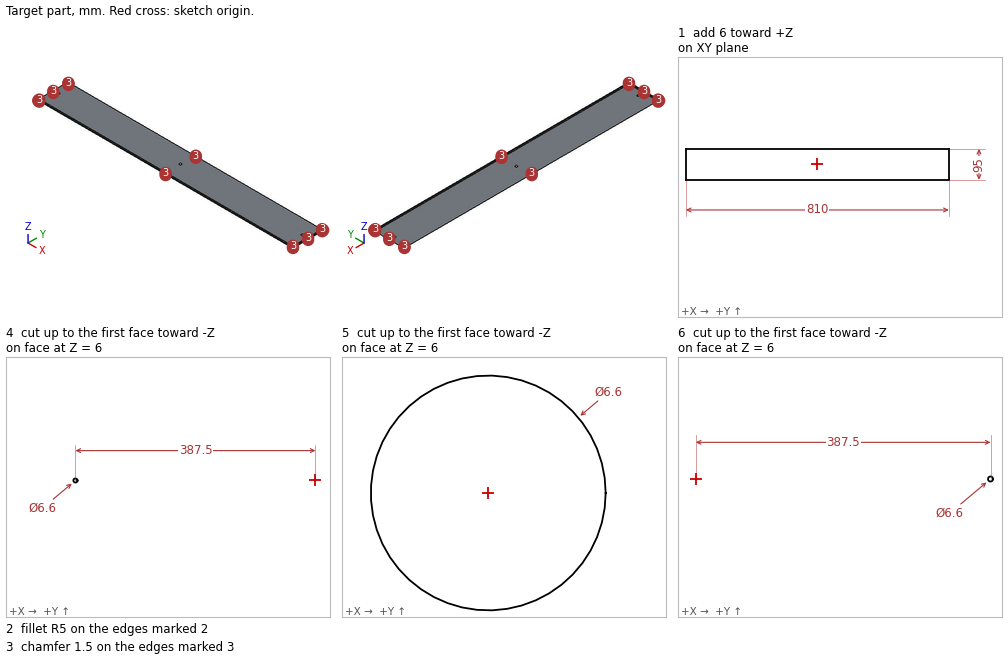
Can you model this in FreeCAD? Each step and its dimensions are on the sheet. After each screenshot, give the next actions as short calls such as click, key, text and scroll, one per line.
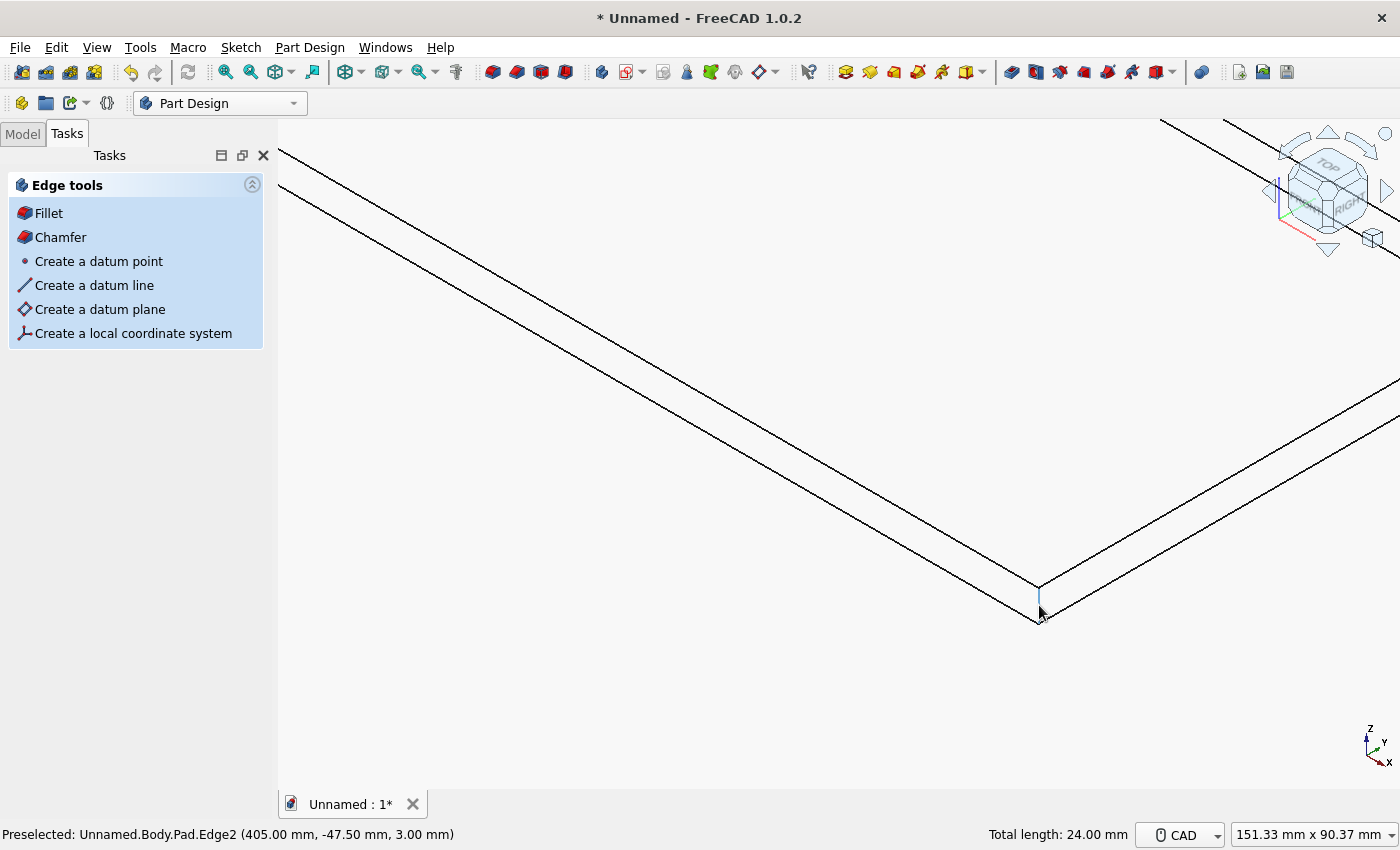
key(v)
key(1)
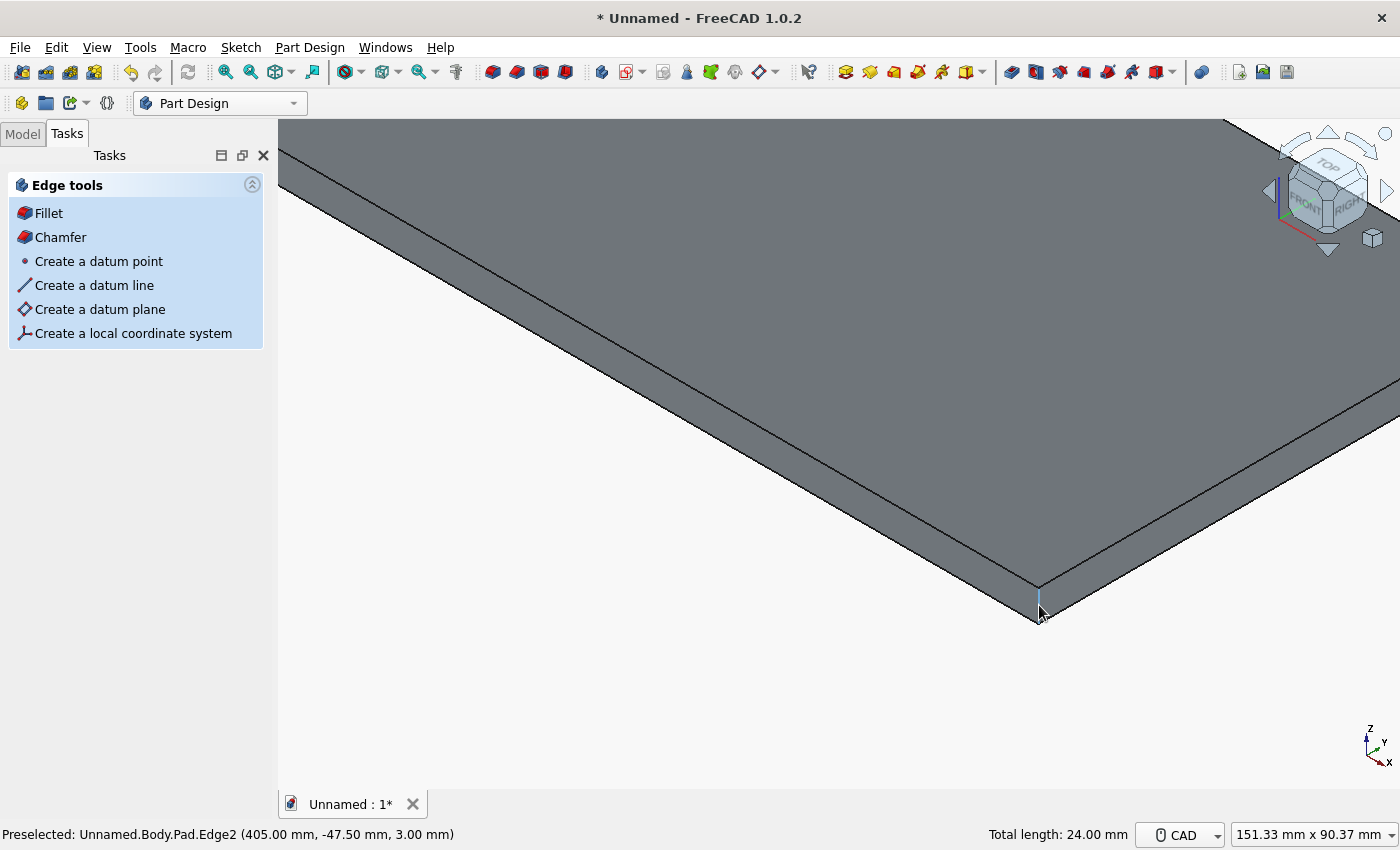
click(494, 72)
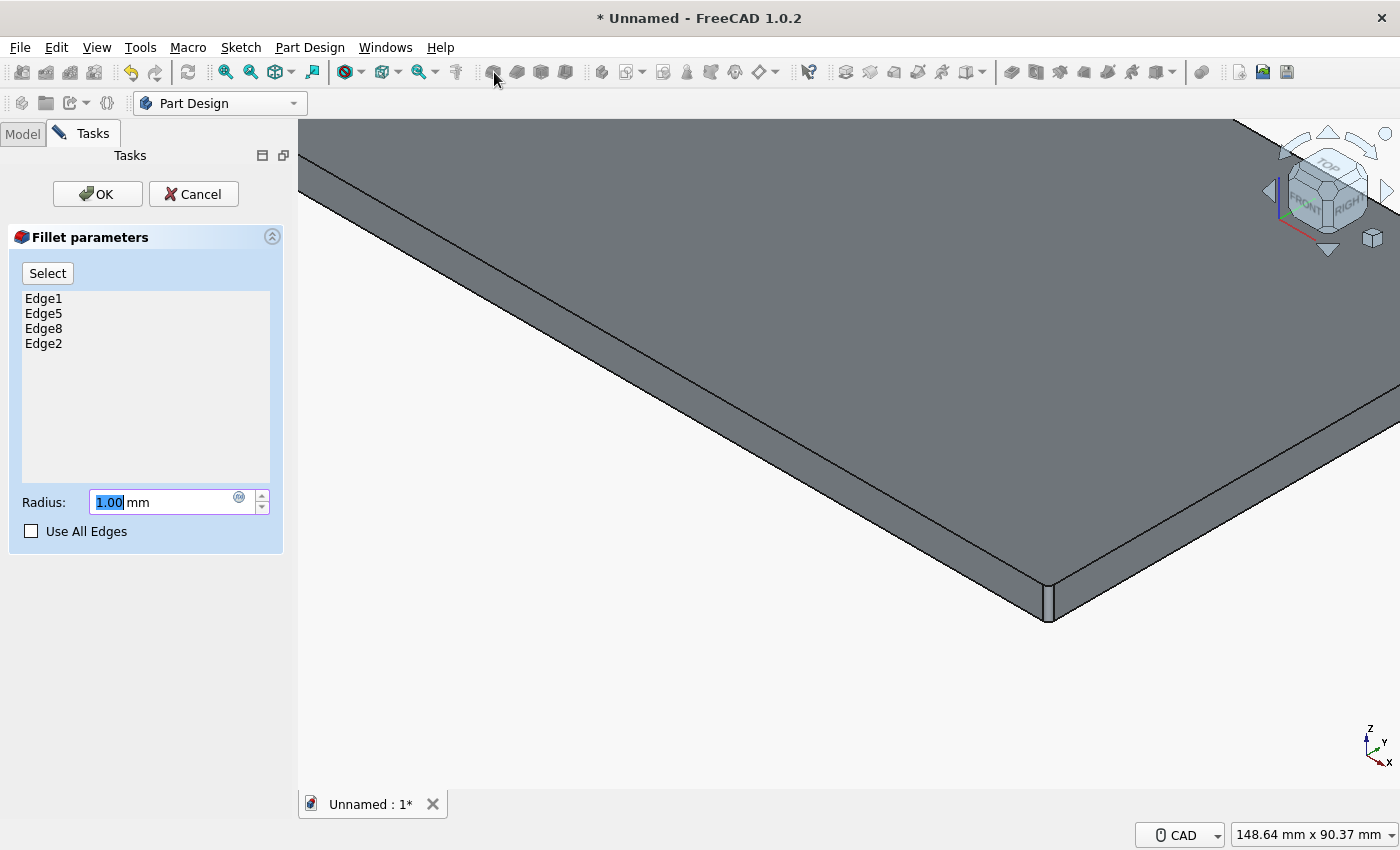
text(5)
key(Tab)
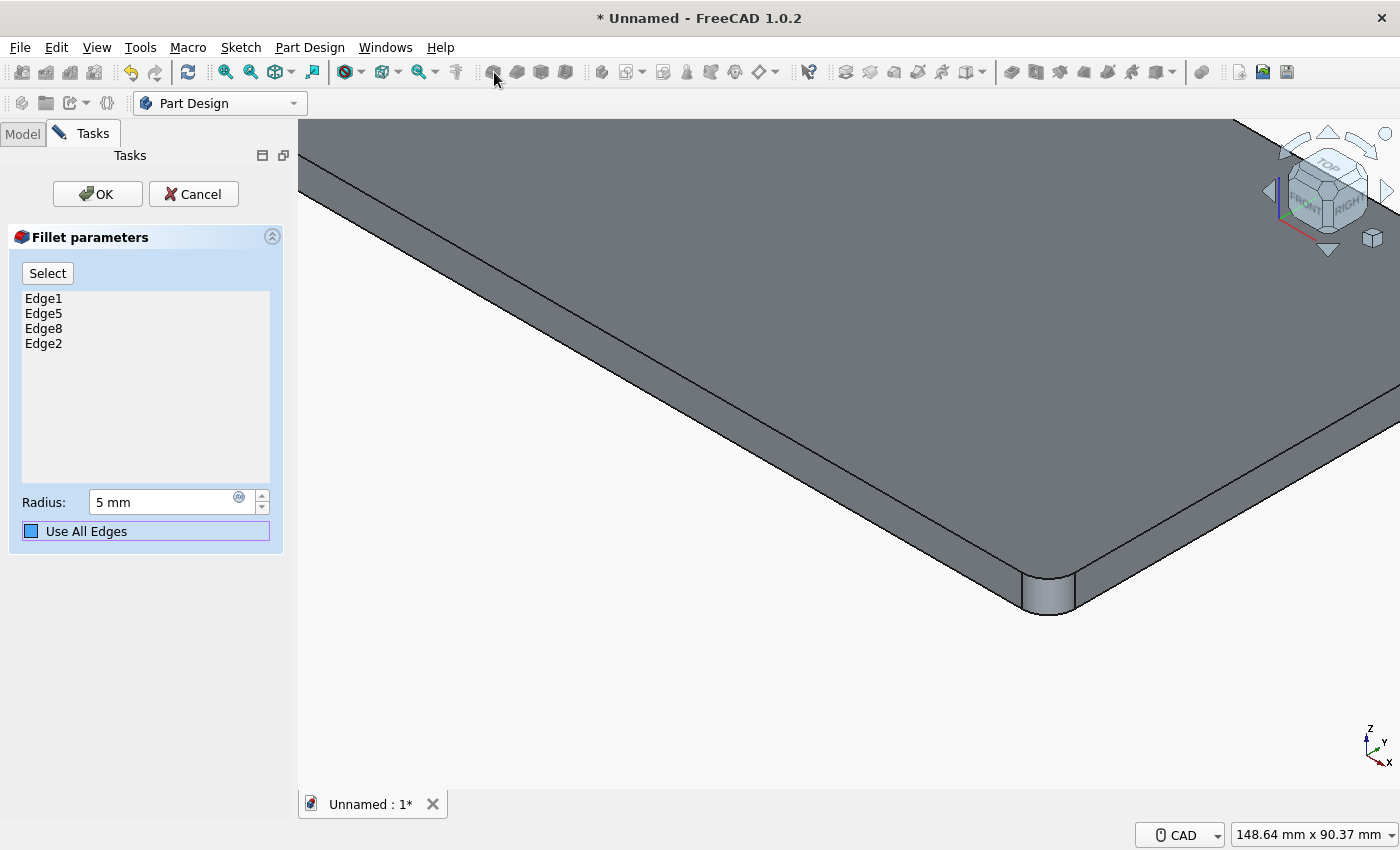
click(98, 194)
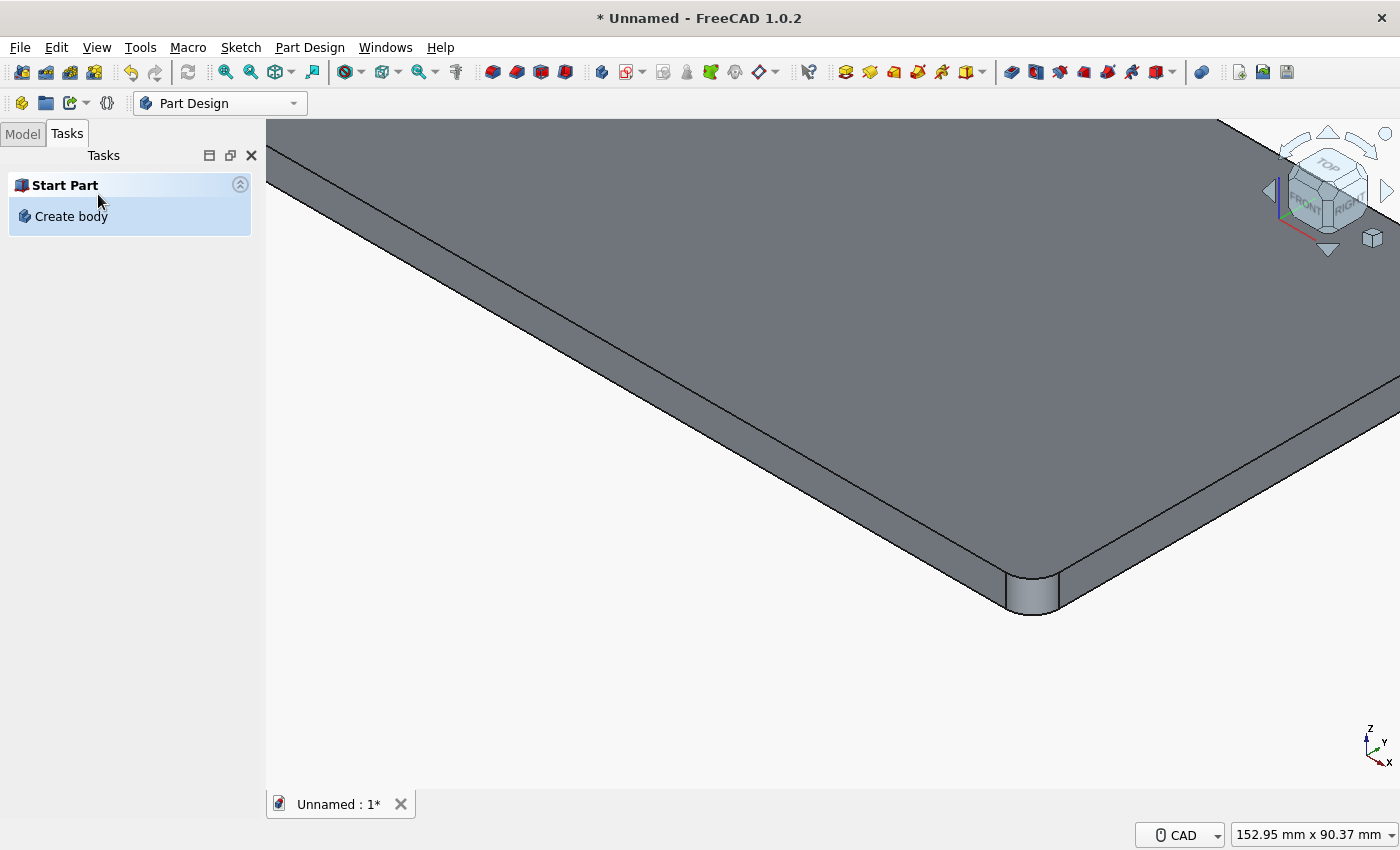
key(v)
key(f)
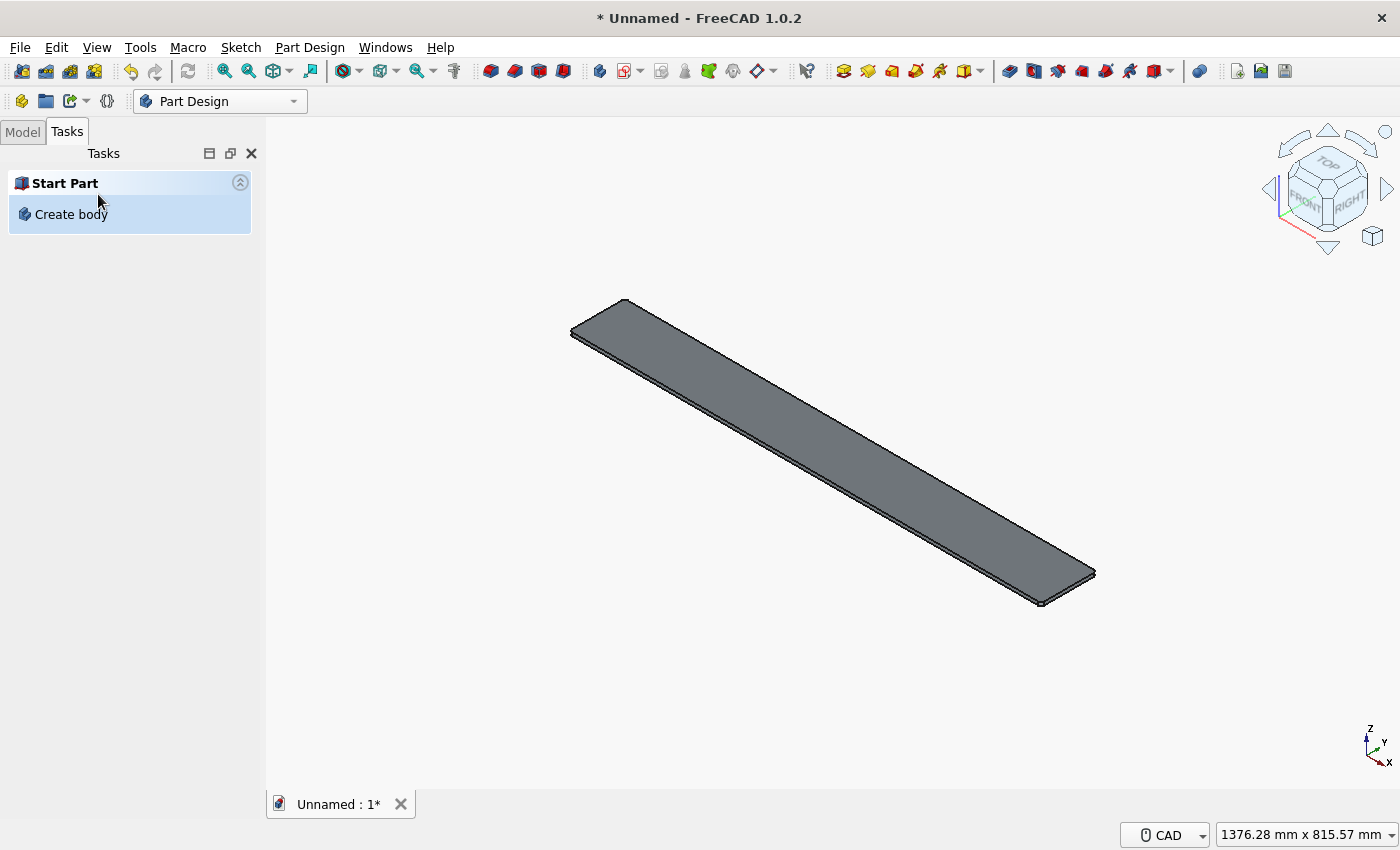
click(1035, 567)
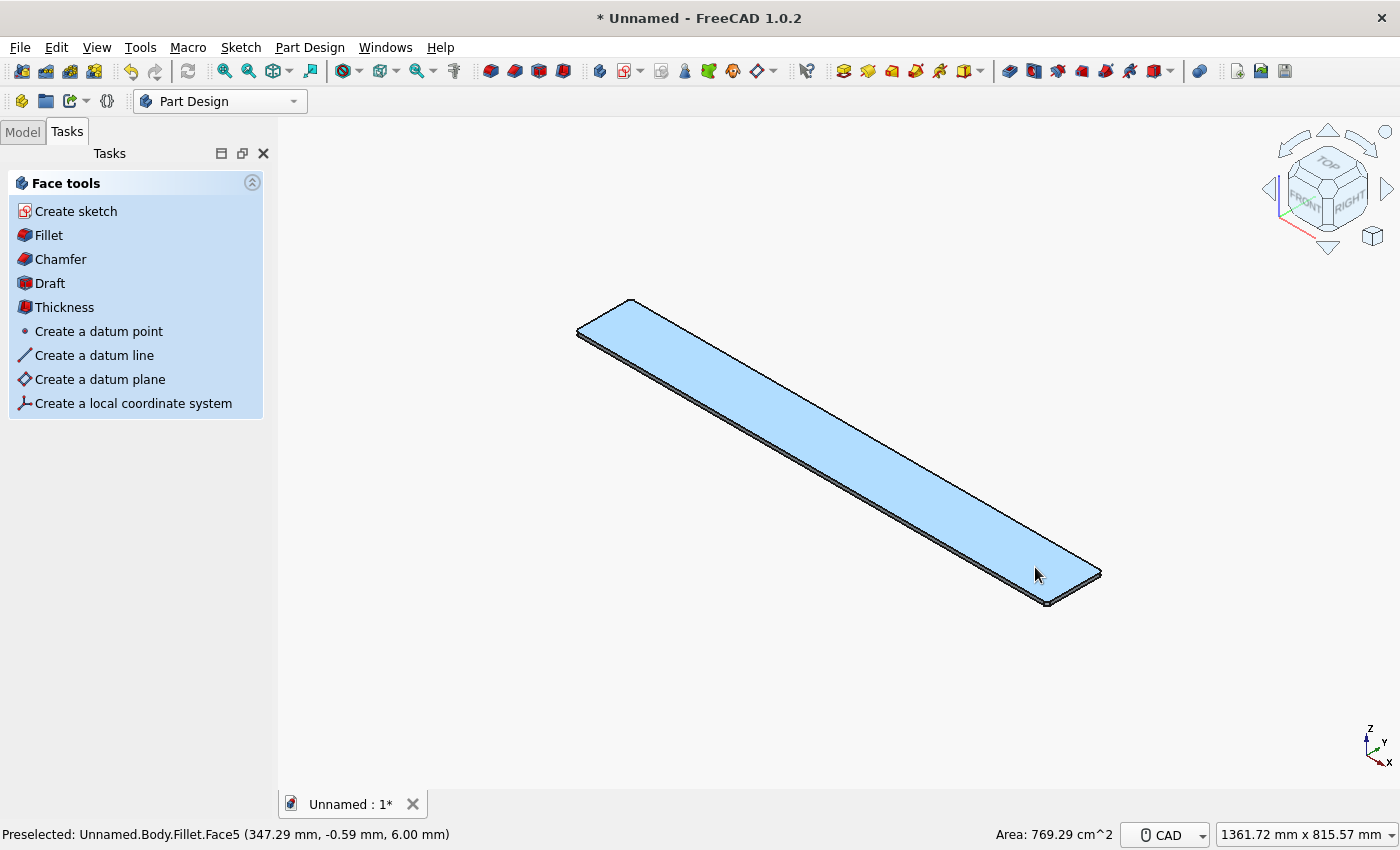
key(2)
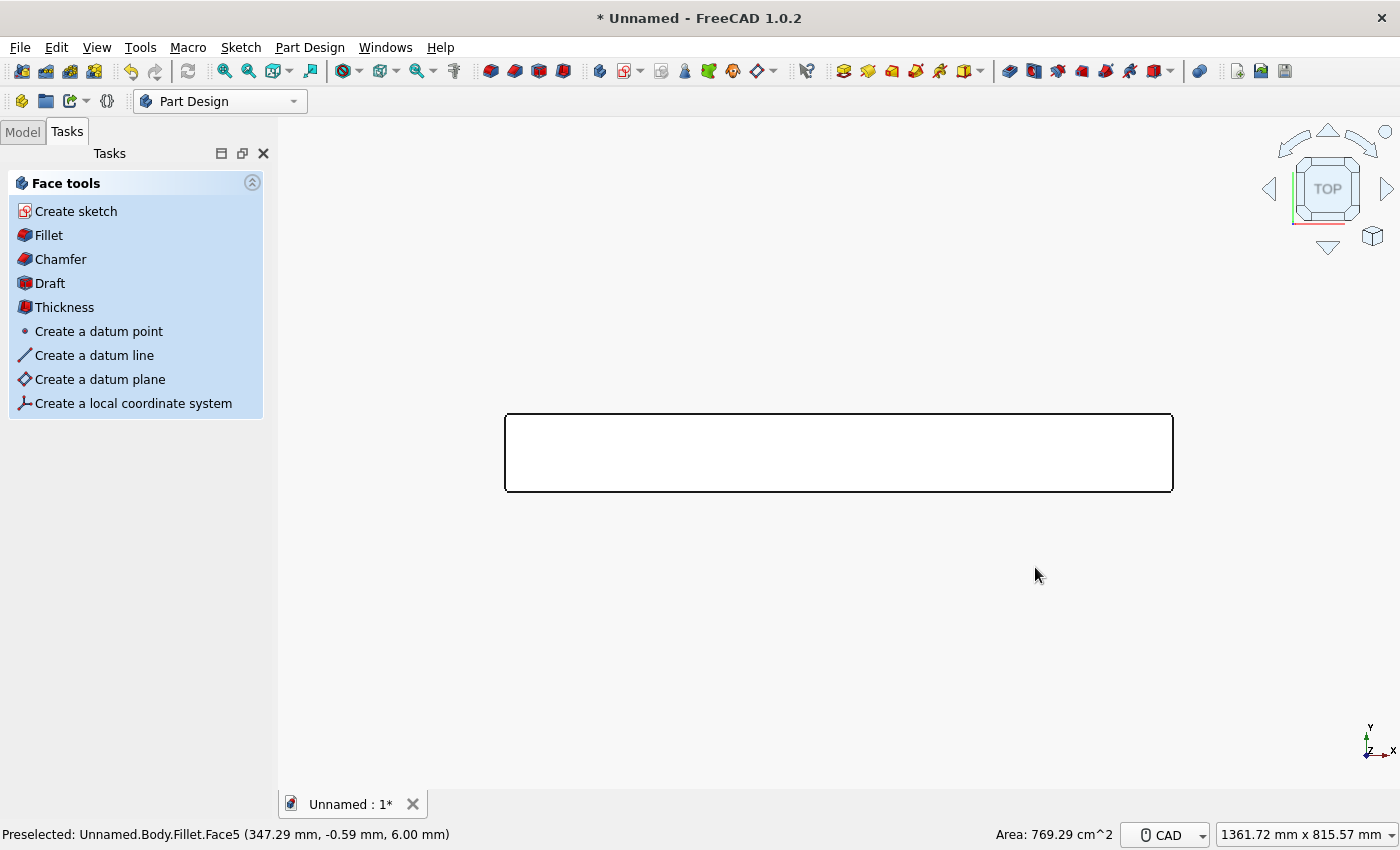
key(0)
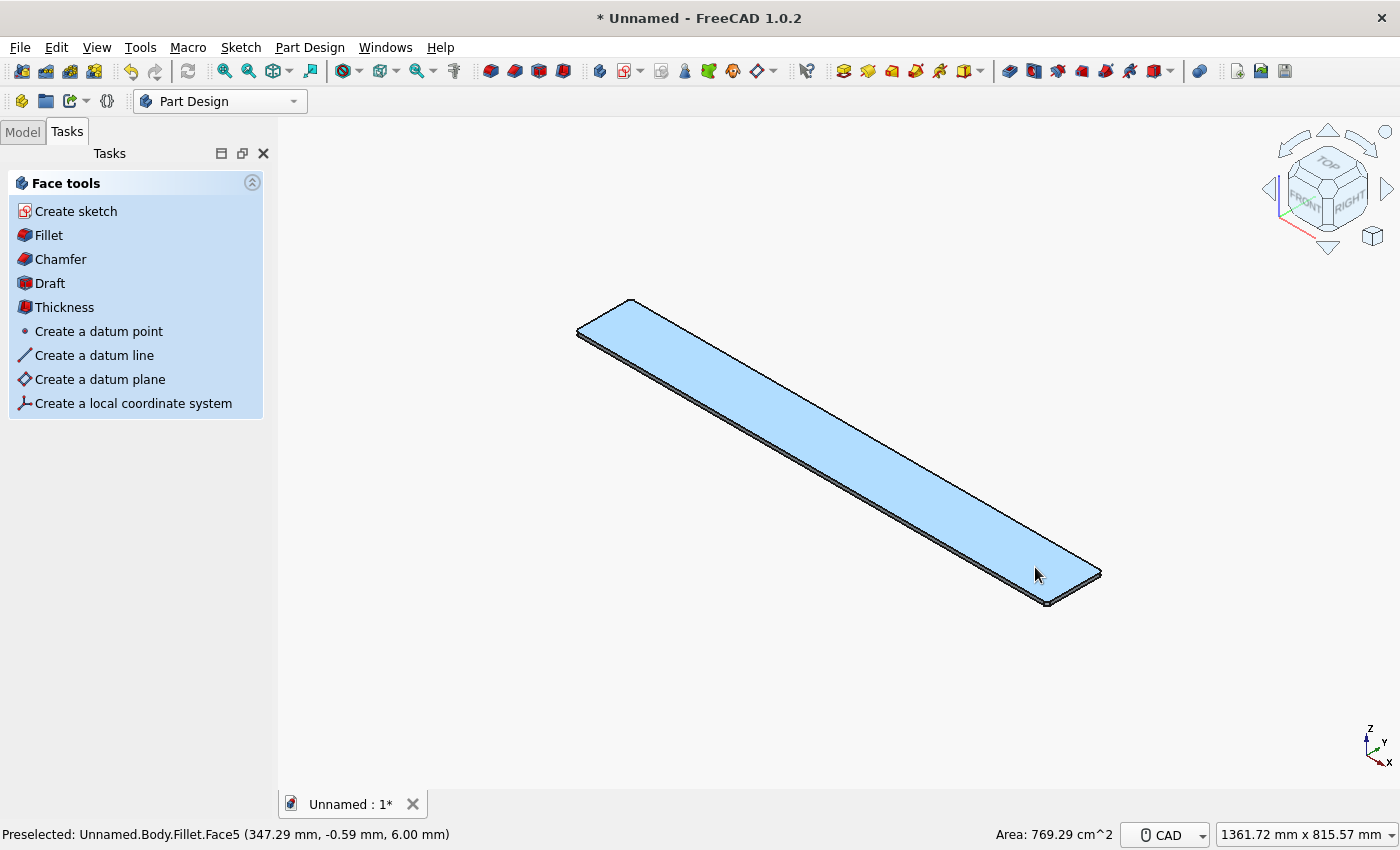
key(1)